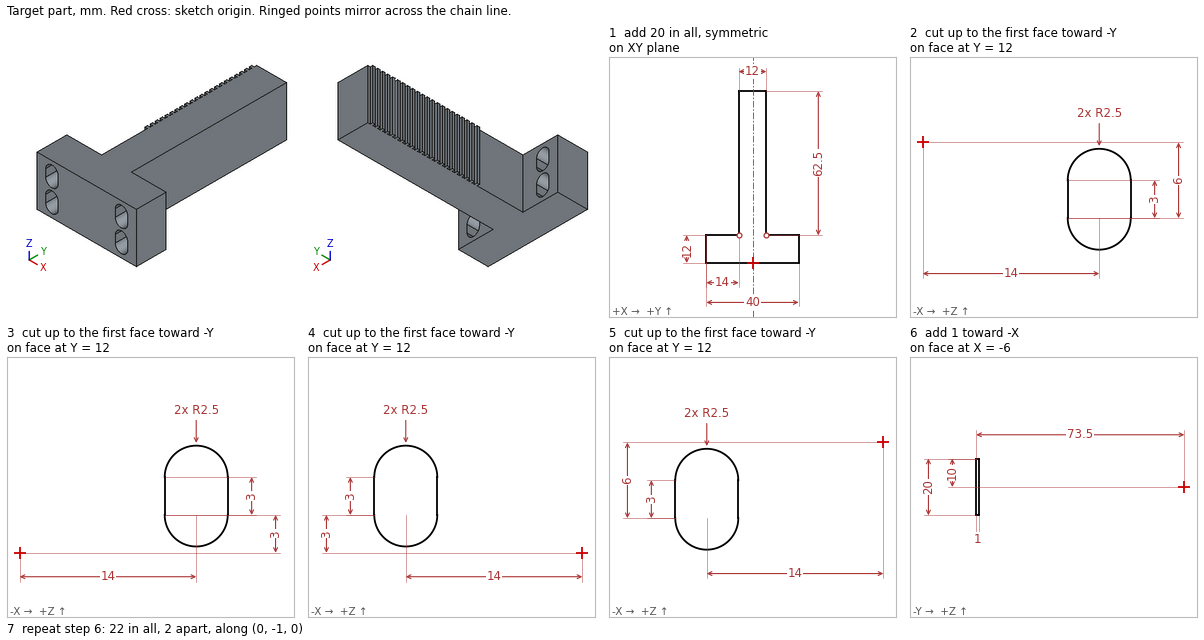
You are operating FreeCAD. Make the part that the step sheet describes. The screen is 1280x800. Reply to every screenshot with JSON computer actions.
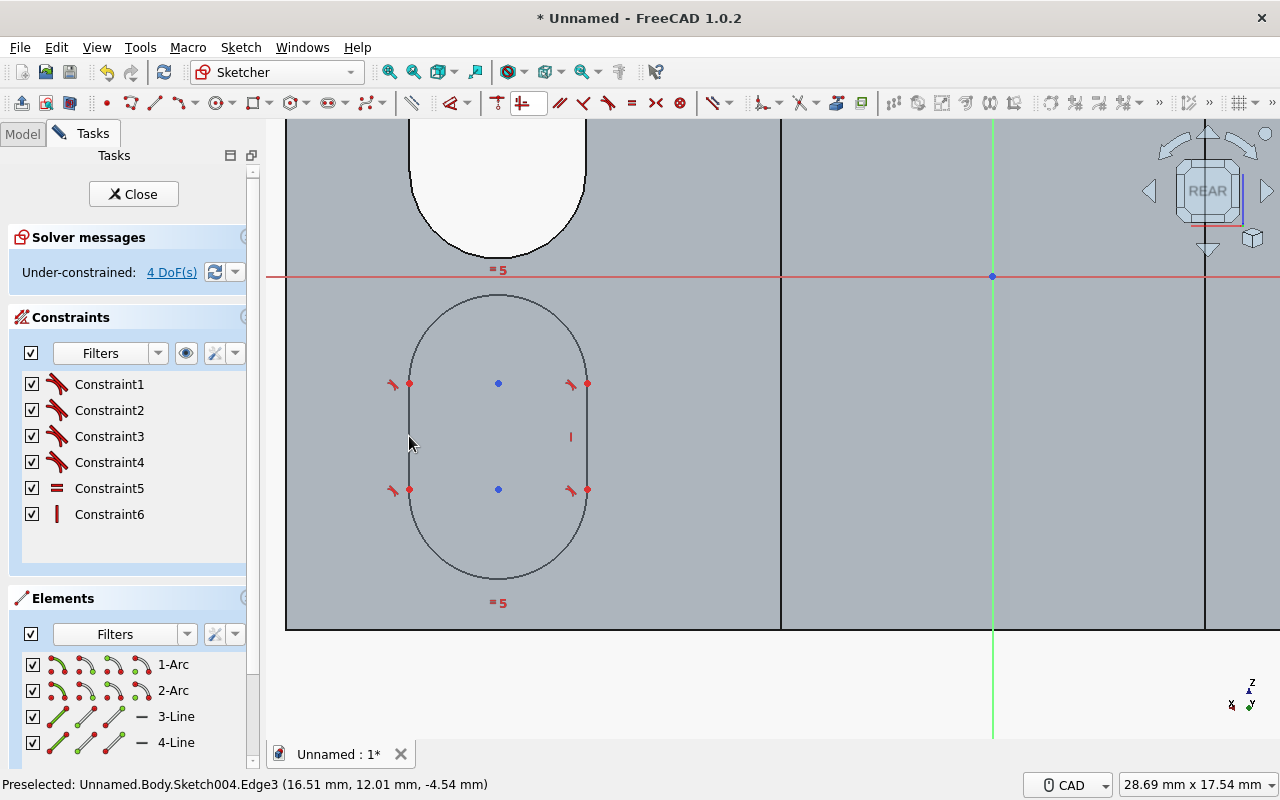
{"action": "left_click", "coordinate": [450, 104]}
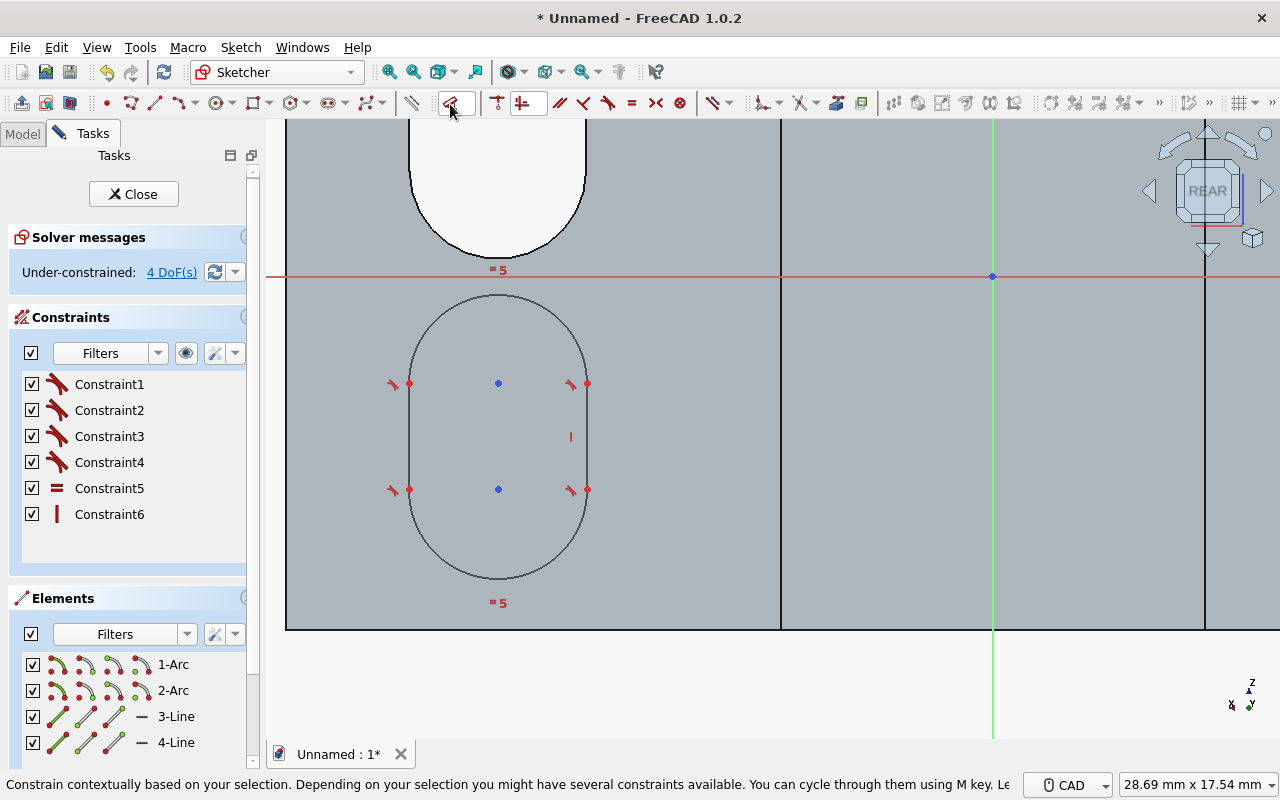
{"action": "left_click", "coordinate": [446, 562]}
{"action": "left_click", "coordinate": [427, 588]}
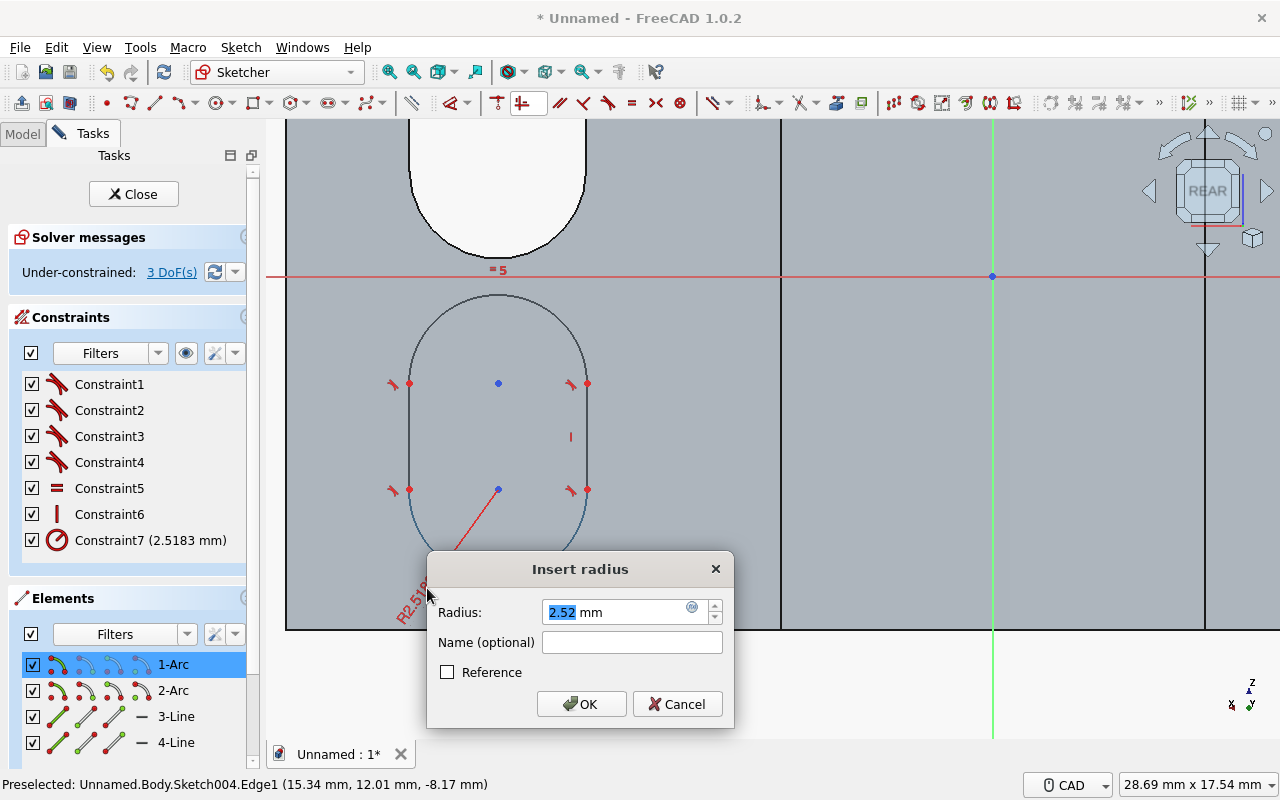
{"action": "type", "text": "2.5"}
{"action": "key", "text": "Return"}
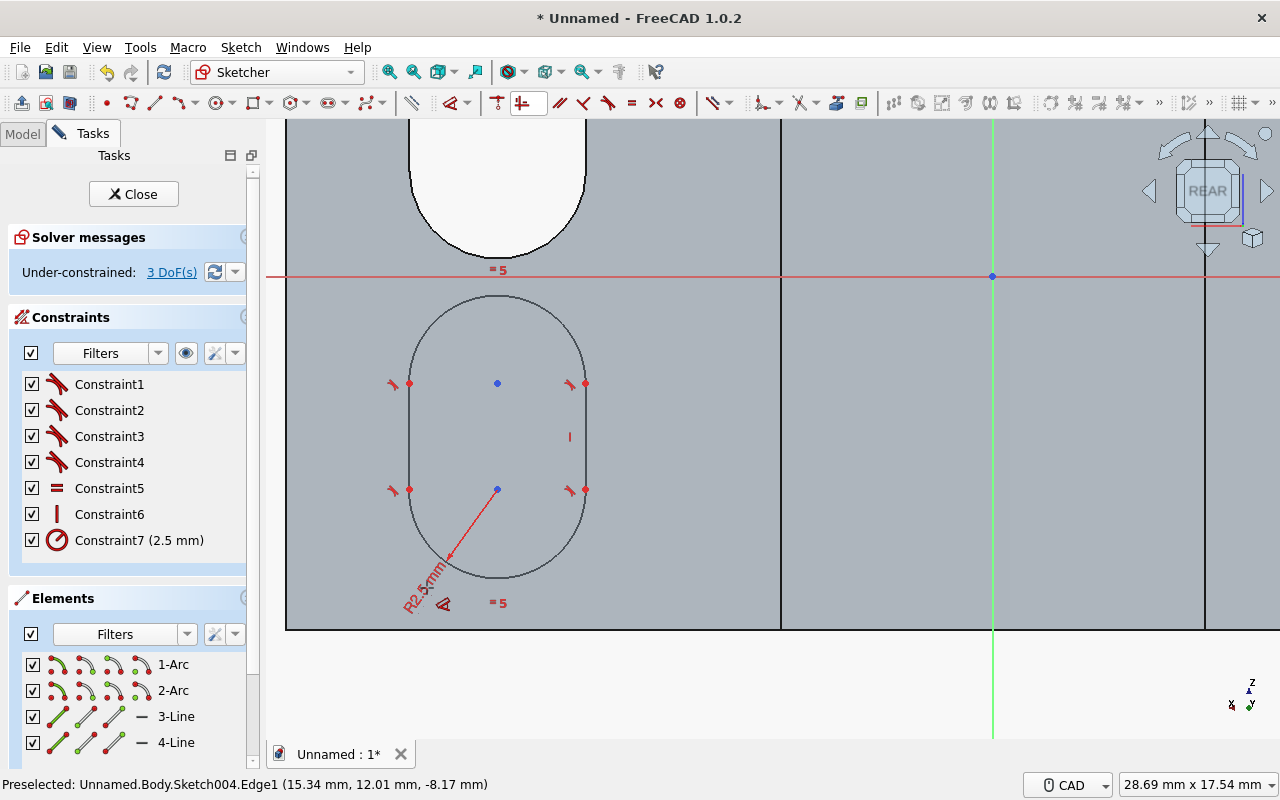
{"action": "left_click", "coordinate": [409, 458]}
{"action": "left_click", "coordinate": [375, 437]}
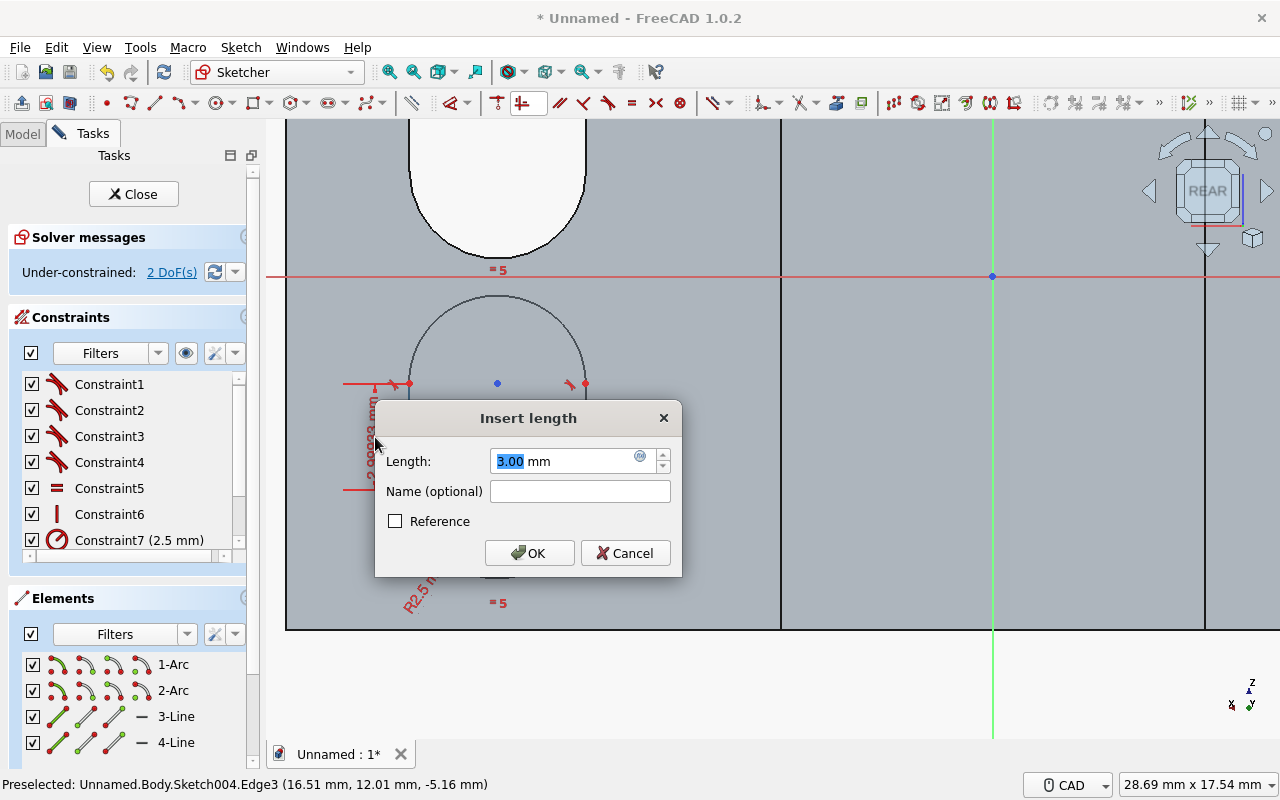
{"action": "type", "text": "3"}
{"action": "key", "text": "Return"}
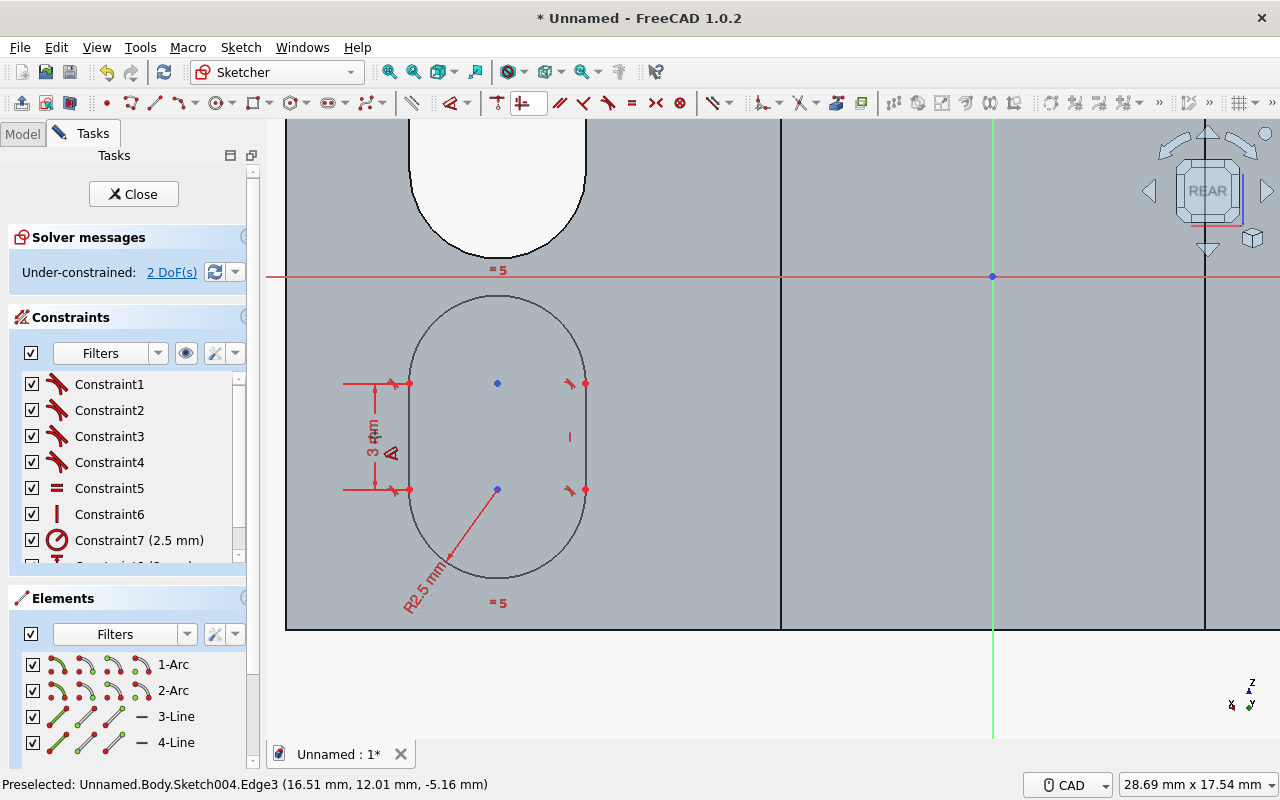
{"action": "left_click", "coordinate": [409, 490]}
{"action": "left_click", "coordinate": [375, 383]}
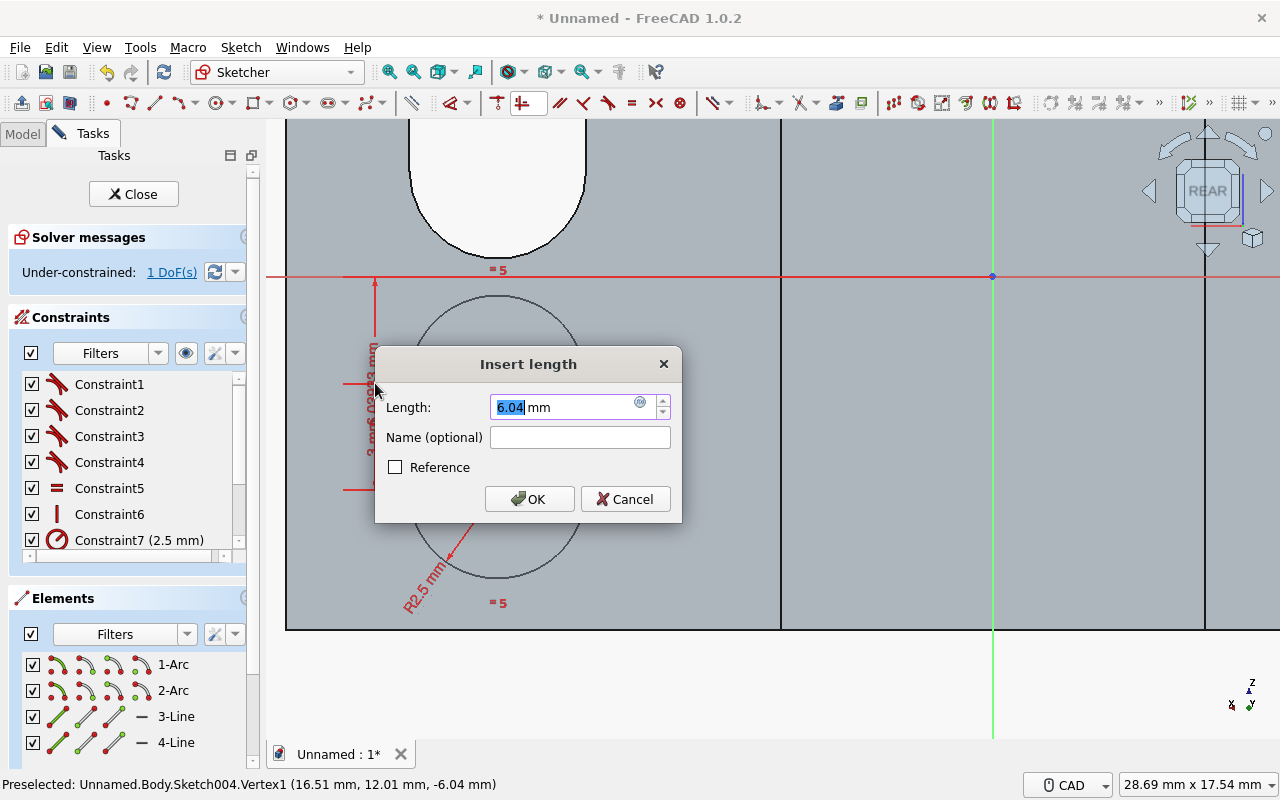
{"action": "type", "text": "6"}
{"action": "key", "text": "Return"}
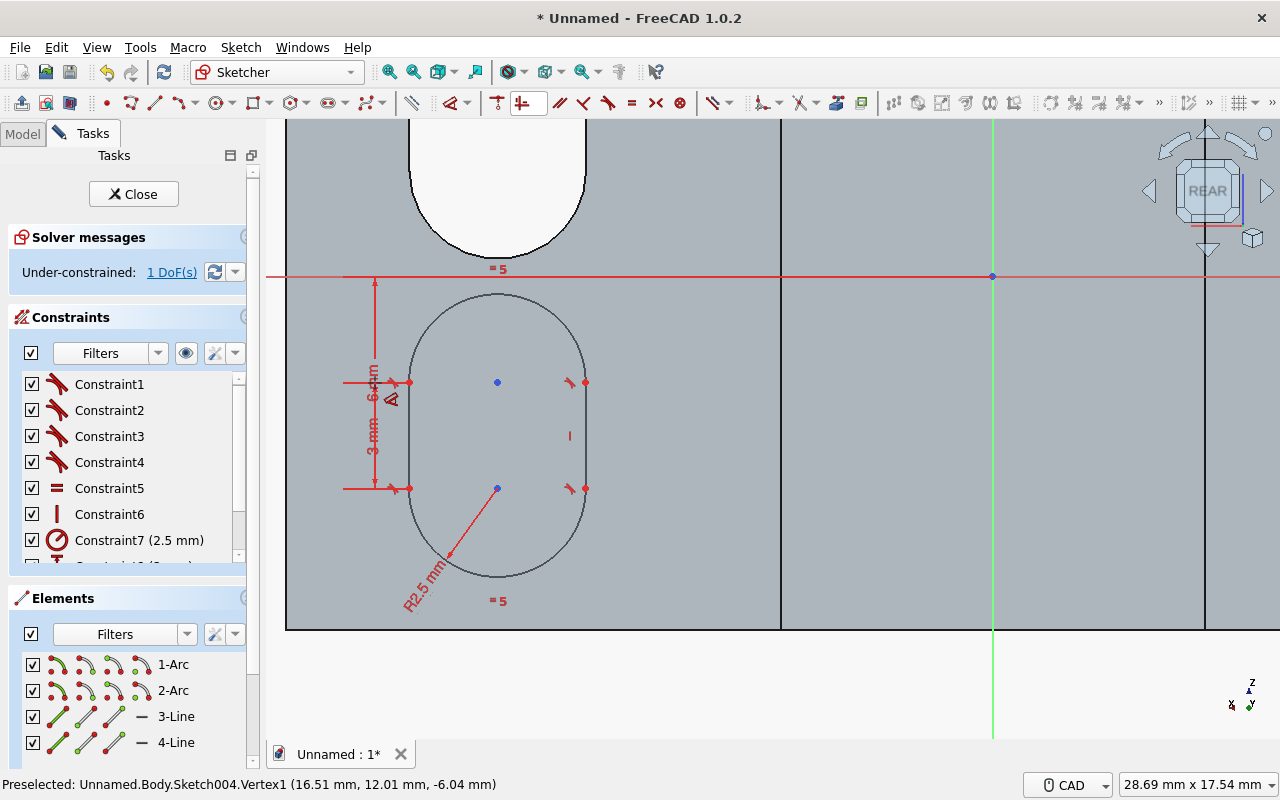
{"action": "left_click", "coordinate": [497, 489]}
{"action": "left_click", "coordinate": [745, 243]}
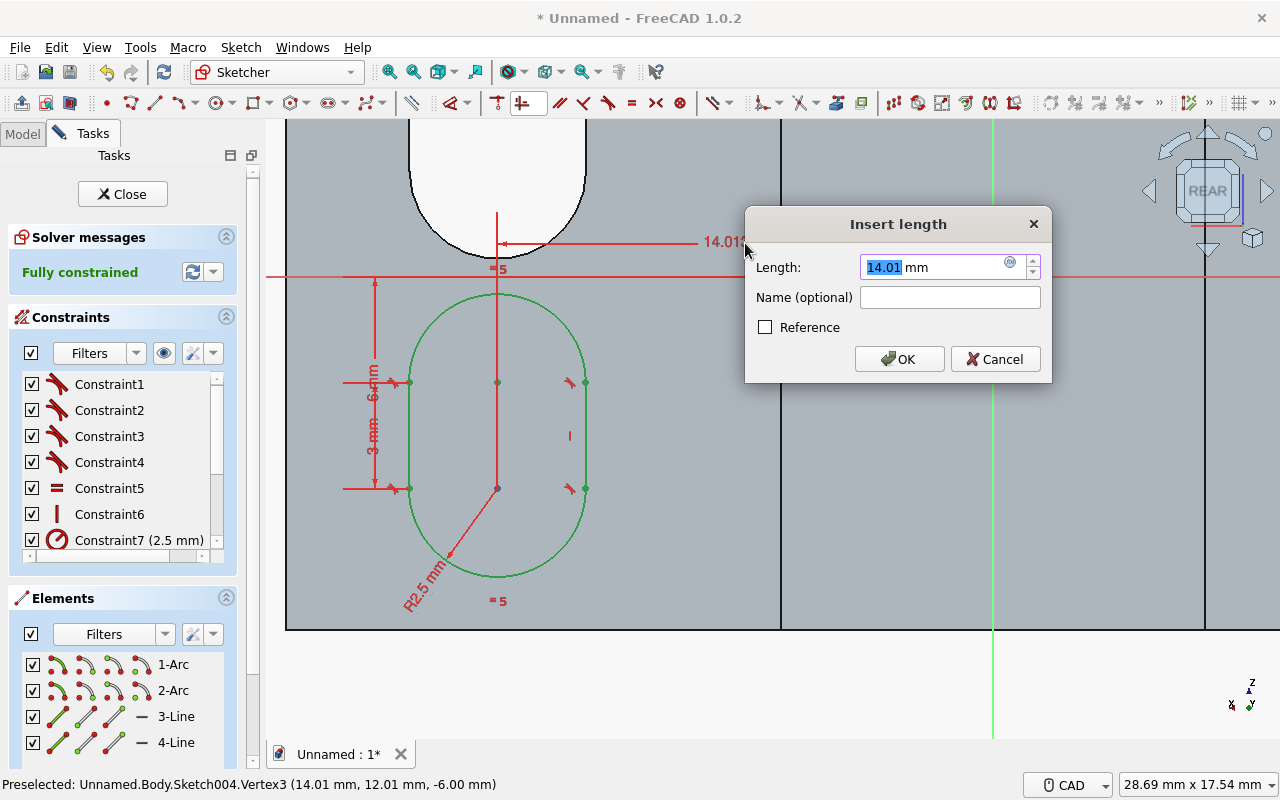
{"action": "type", "text": "14"}
{"action": "key", "text": "Return"}
{"action": "key", "text": "Escape"}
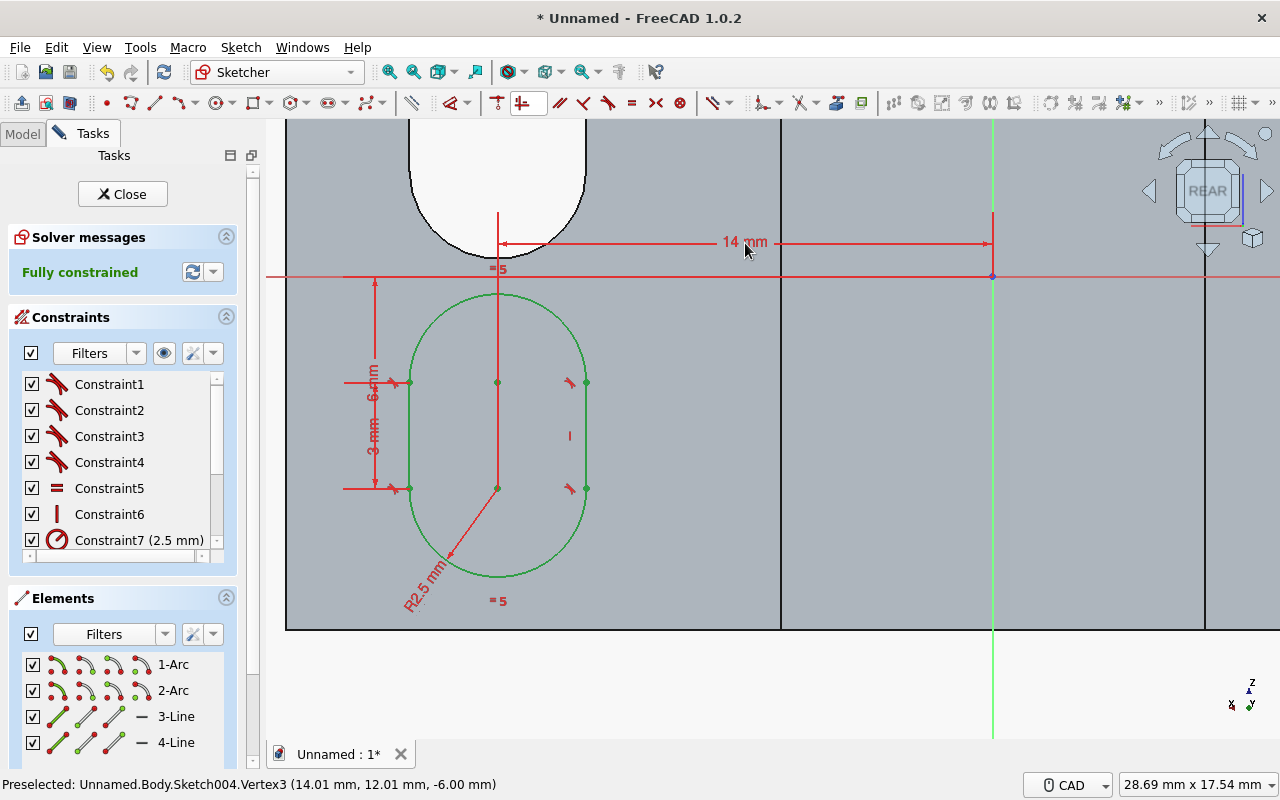
{"action": "left_click", "coordinate": [123, 194]}